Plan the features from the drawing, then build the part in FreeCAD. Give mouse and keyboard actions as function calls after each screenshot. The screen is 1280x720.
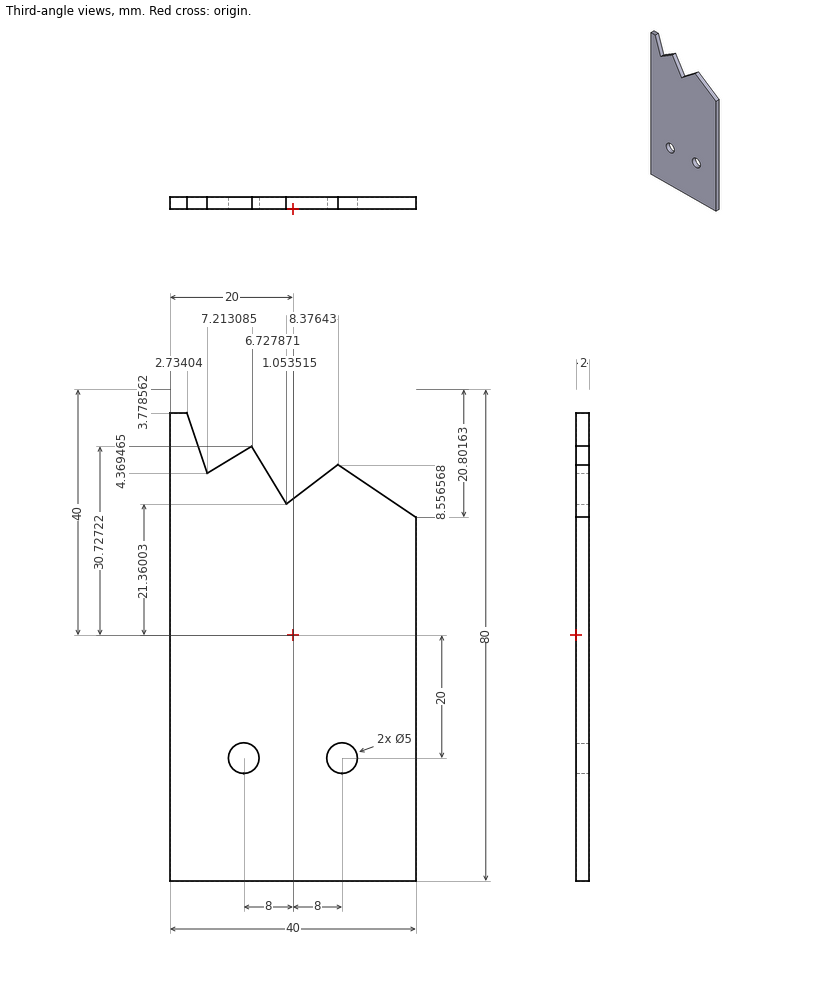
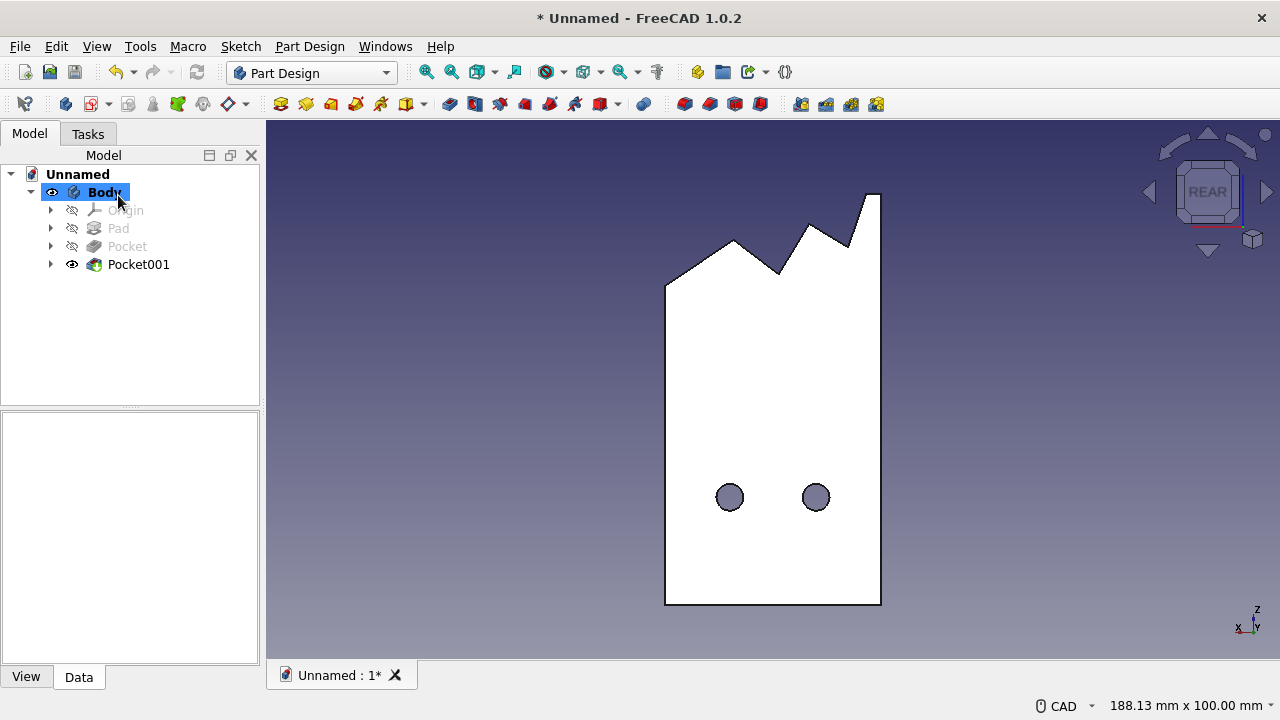
key(0)